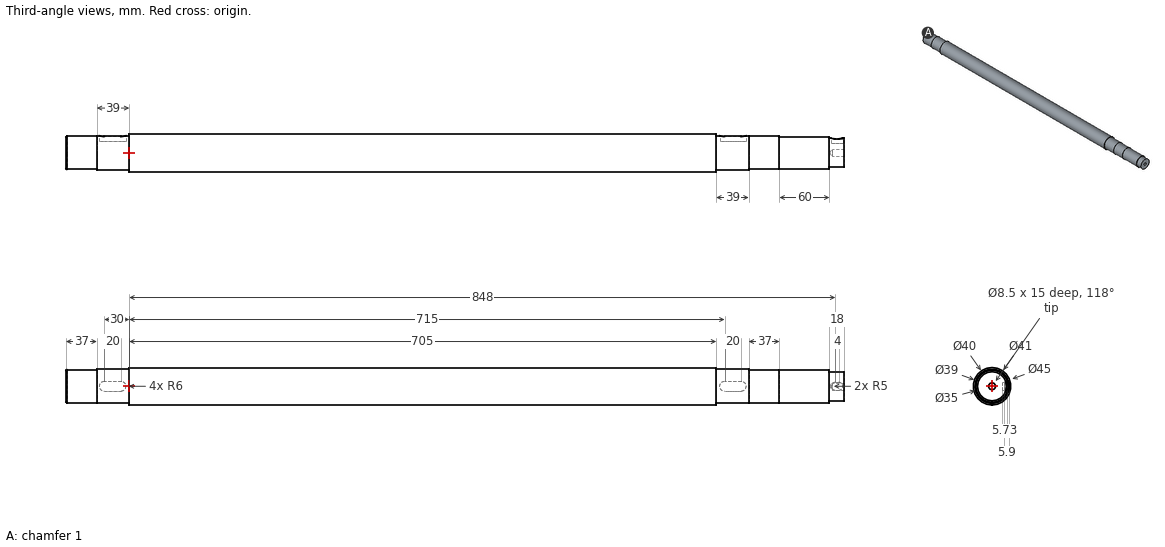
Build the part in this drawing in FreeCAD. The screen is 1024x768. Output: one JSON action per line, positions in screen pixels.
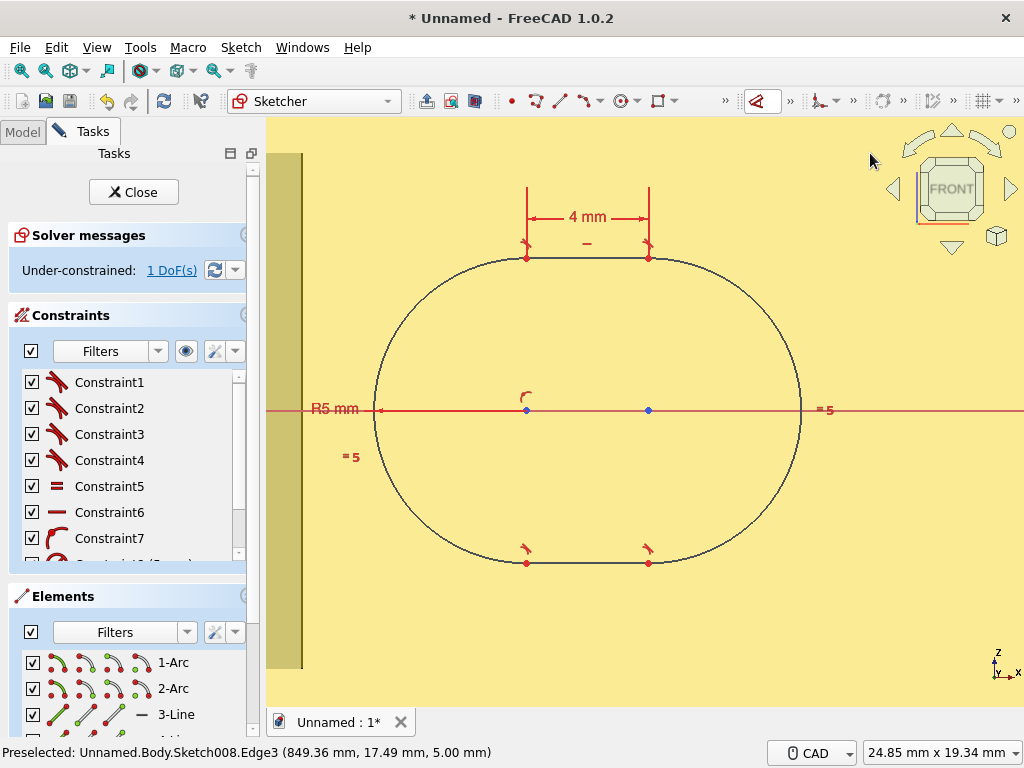
{"action": "left_click", "coordinate": [527, 258]}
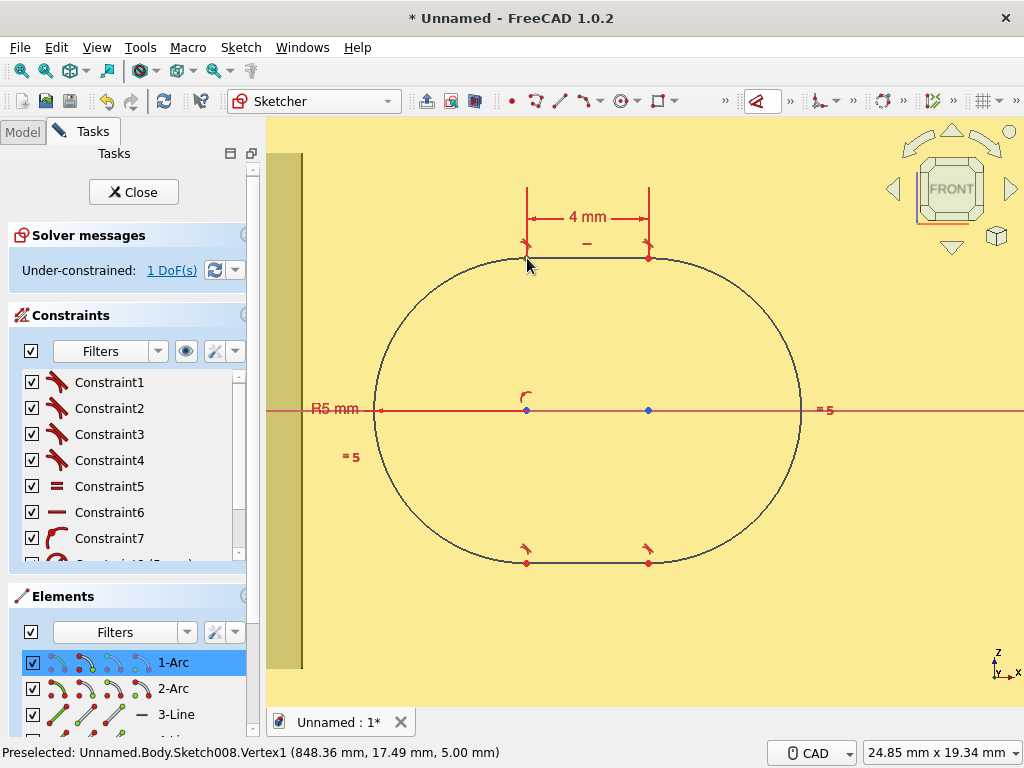
{"action": "key", "text": "l"}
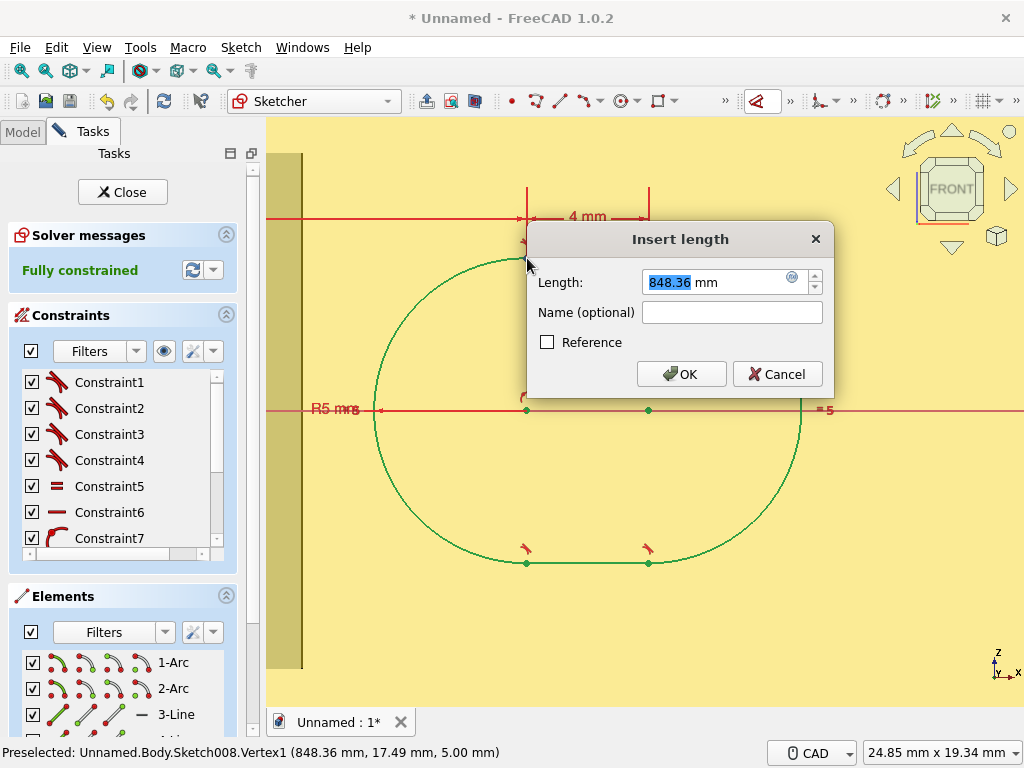
{"action": "type", "text": "848"}
{"action": "key", "text": "Return"}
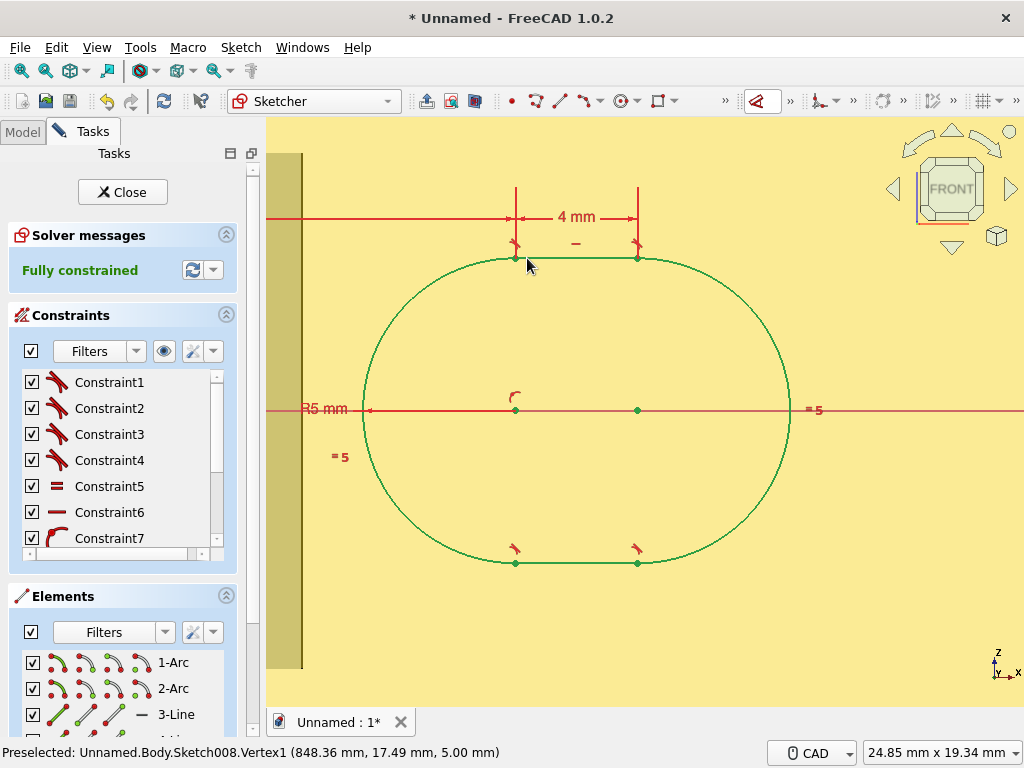
{"action": "left_click", "coordinate": [123, 192]}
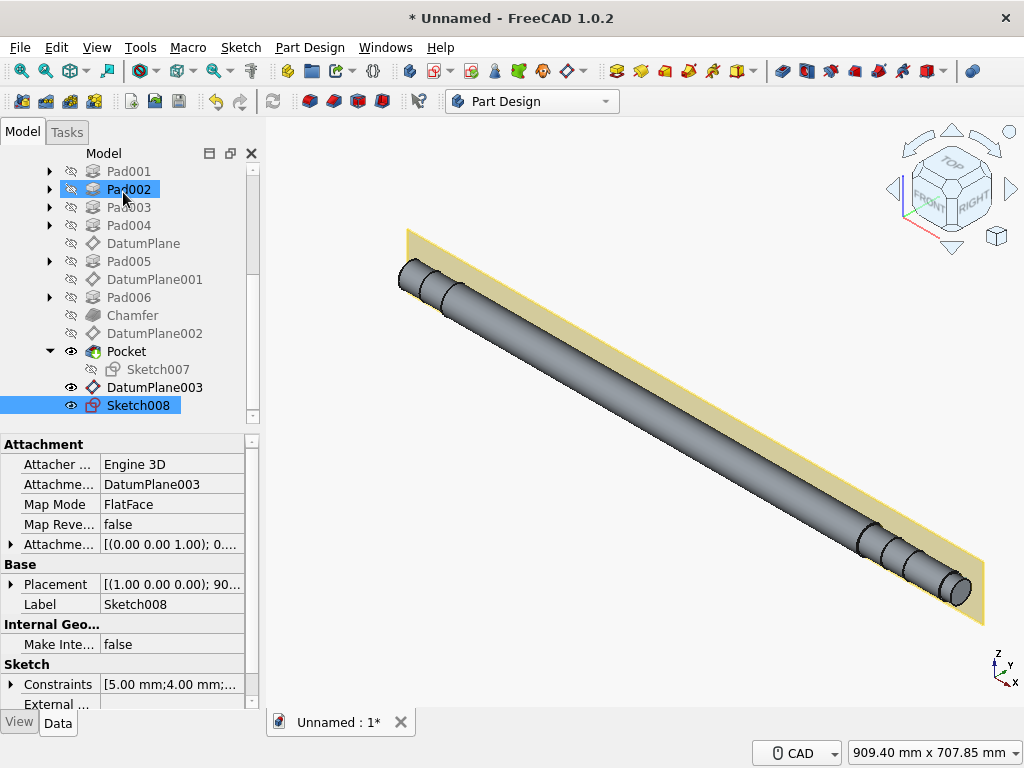
{"action": "left_click", "coordinate": [784, 72]}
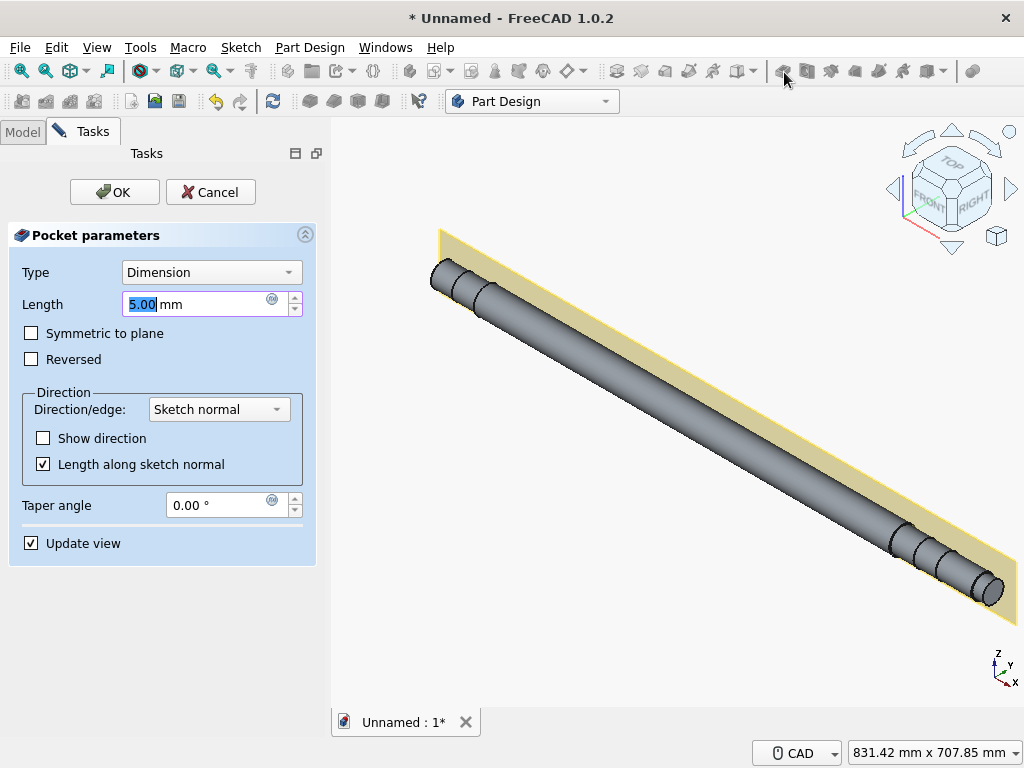
{"action": "type", "text": "5.73"}
{"action": "key", "text": "Tab"}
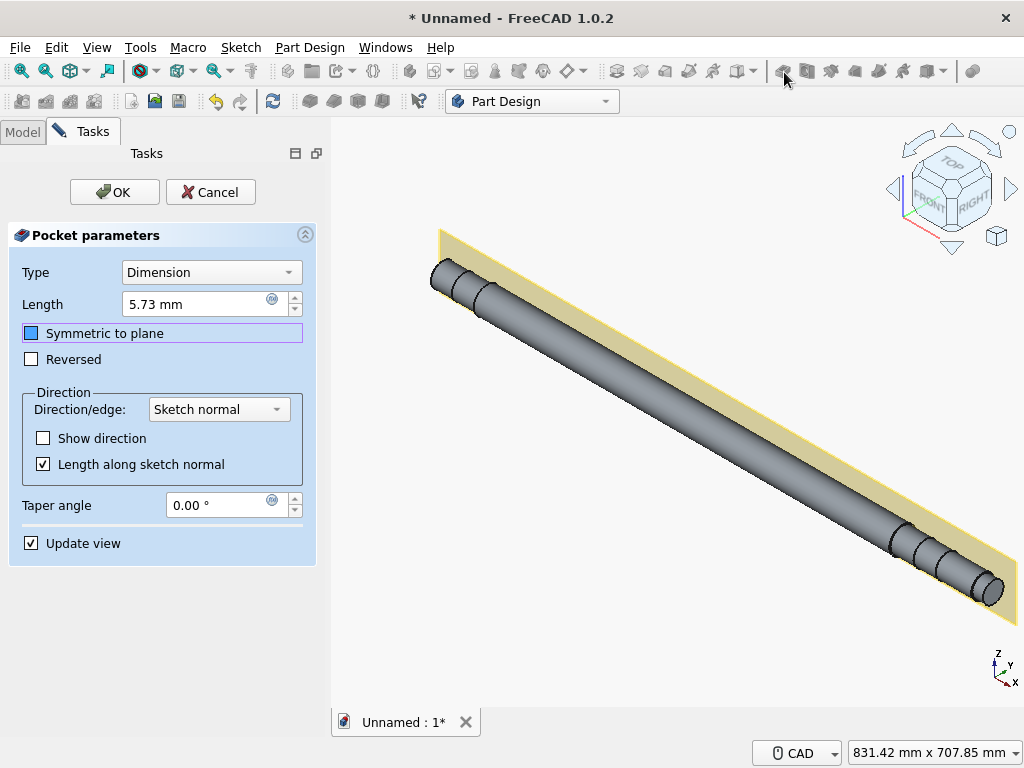
{"action": "left_click", "coordinate": [30, 359]}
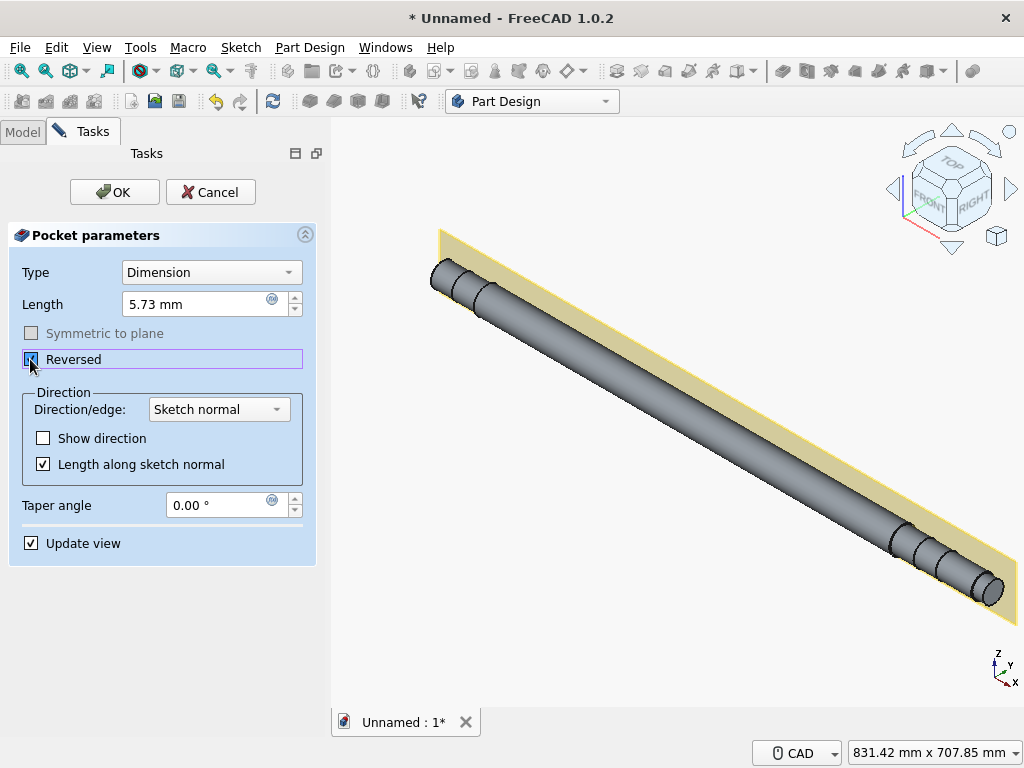
{"action": "left_click", "coordinate": [115, 192]}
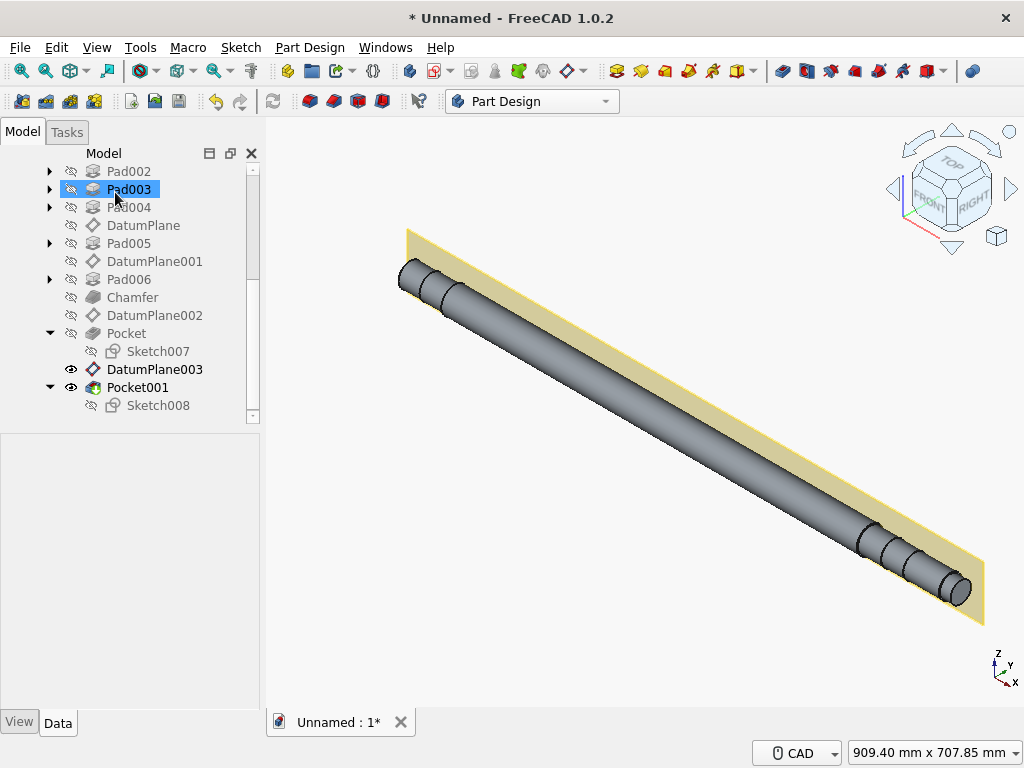
{"action": "left_click", "coordinate": [116, 369]}
{"action": "key", "text": "space"}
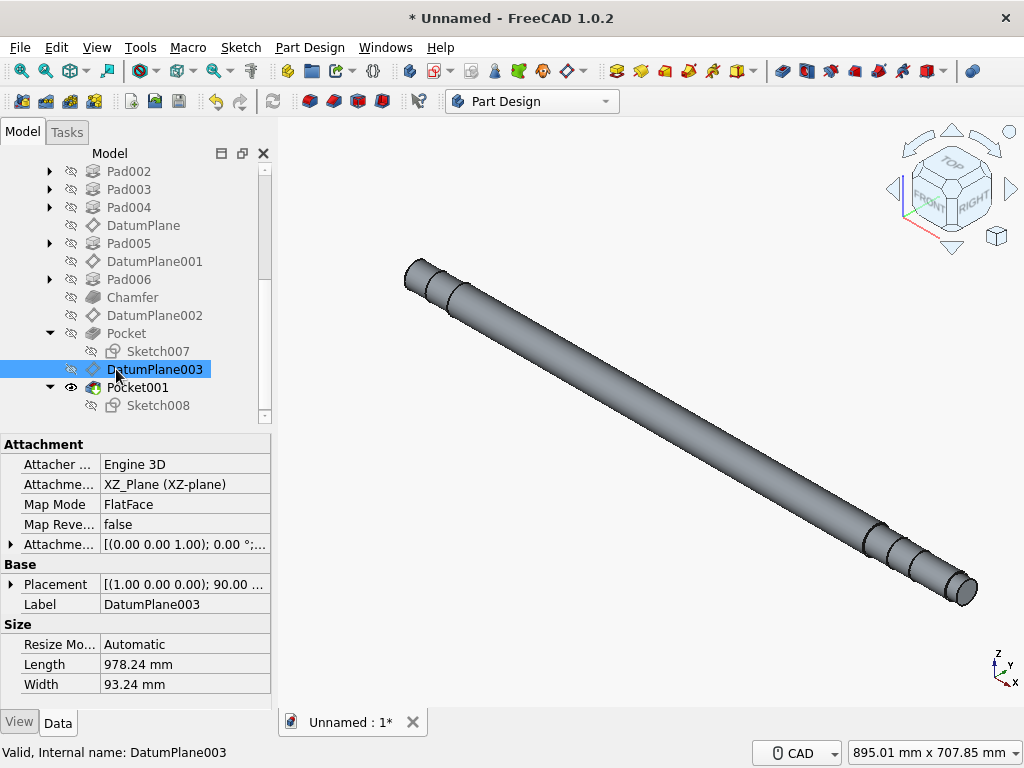
{"action": "key", "text": "3"}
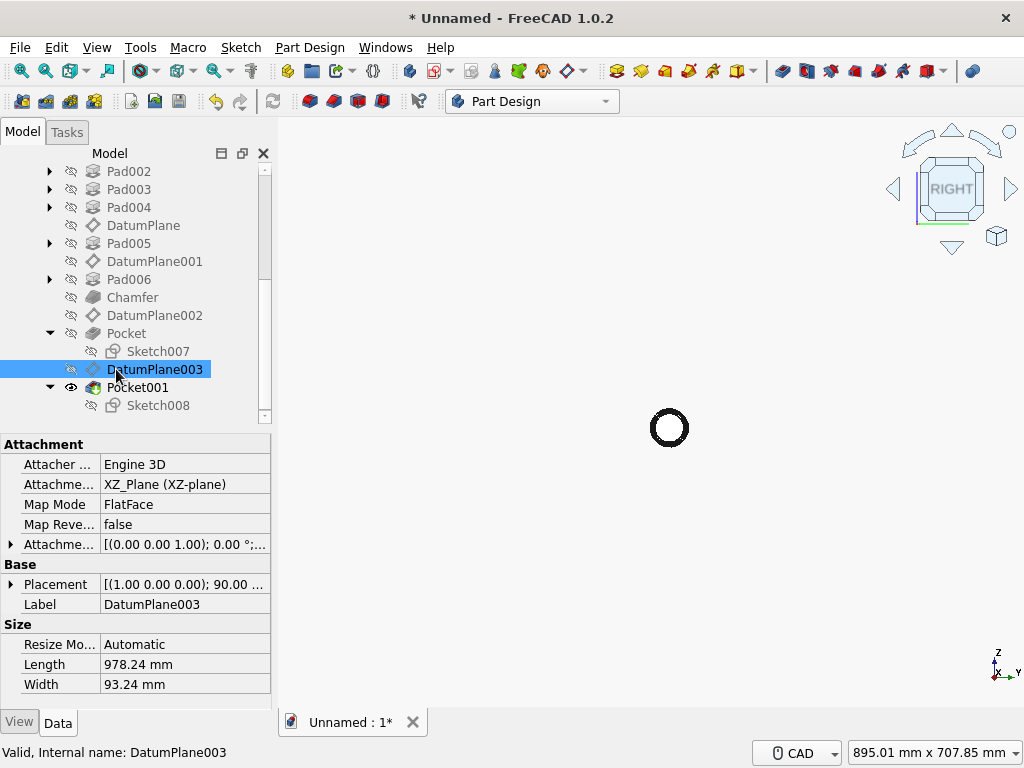
{"action": "left_click", "coordinate": [22, 72]}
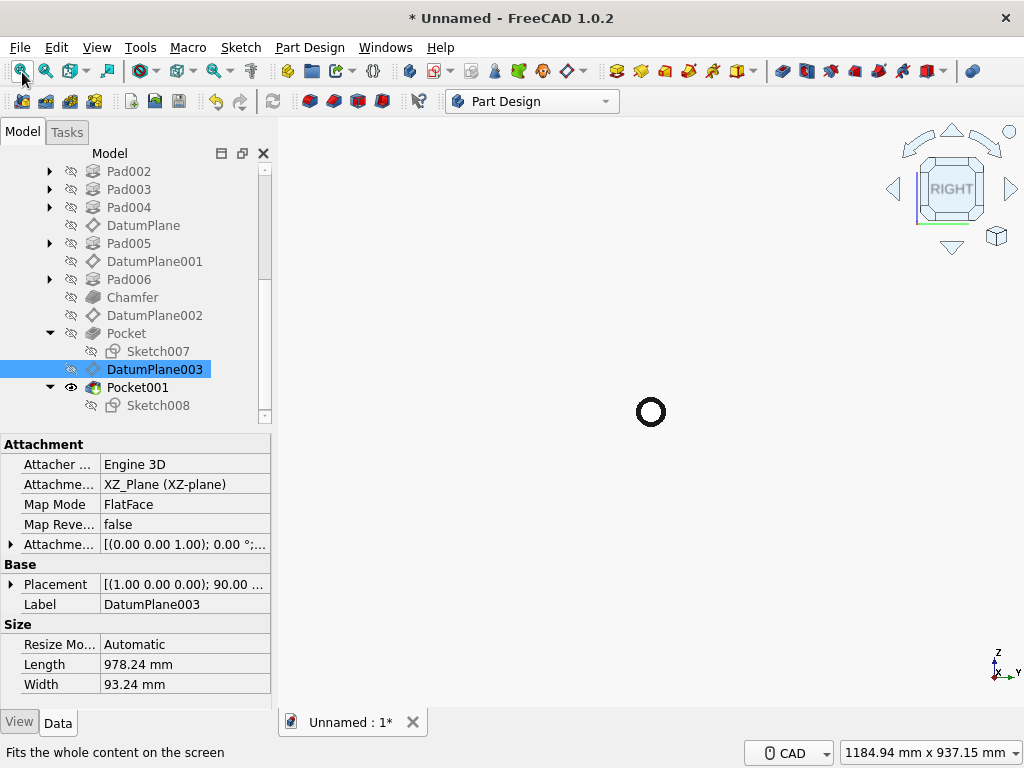
{"action": "left_click", "coordinate": [651, 411]}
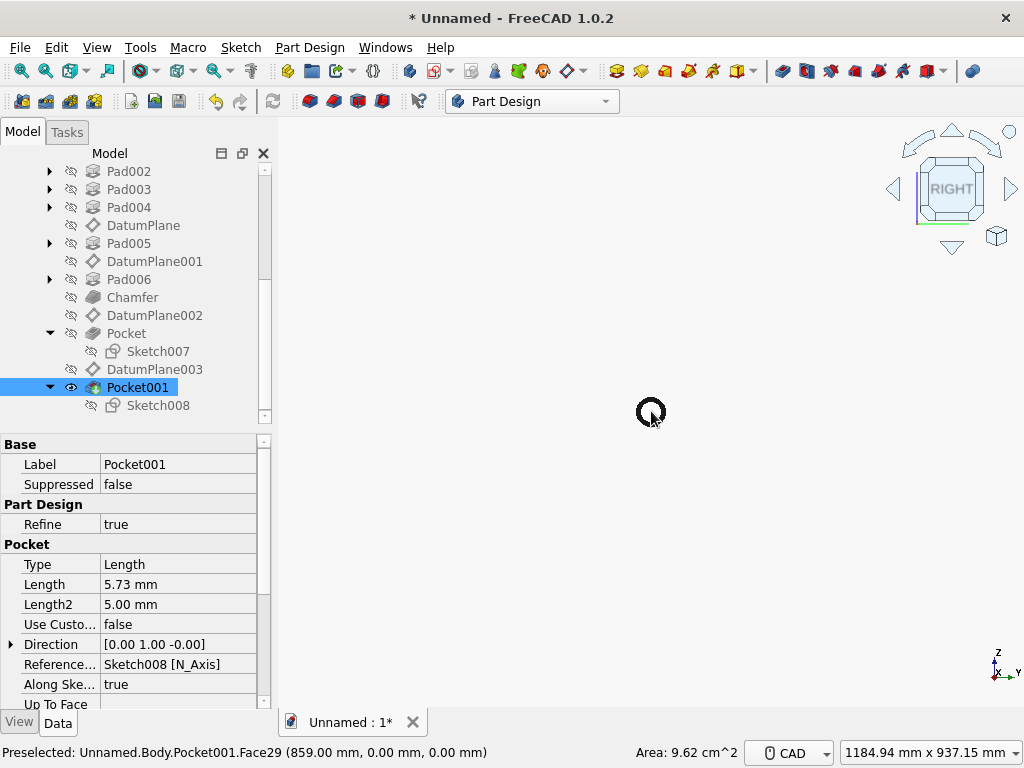
{"action": "left_click", "coordinate": [434, 72]}